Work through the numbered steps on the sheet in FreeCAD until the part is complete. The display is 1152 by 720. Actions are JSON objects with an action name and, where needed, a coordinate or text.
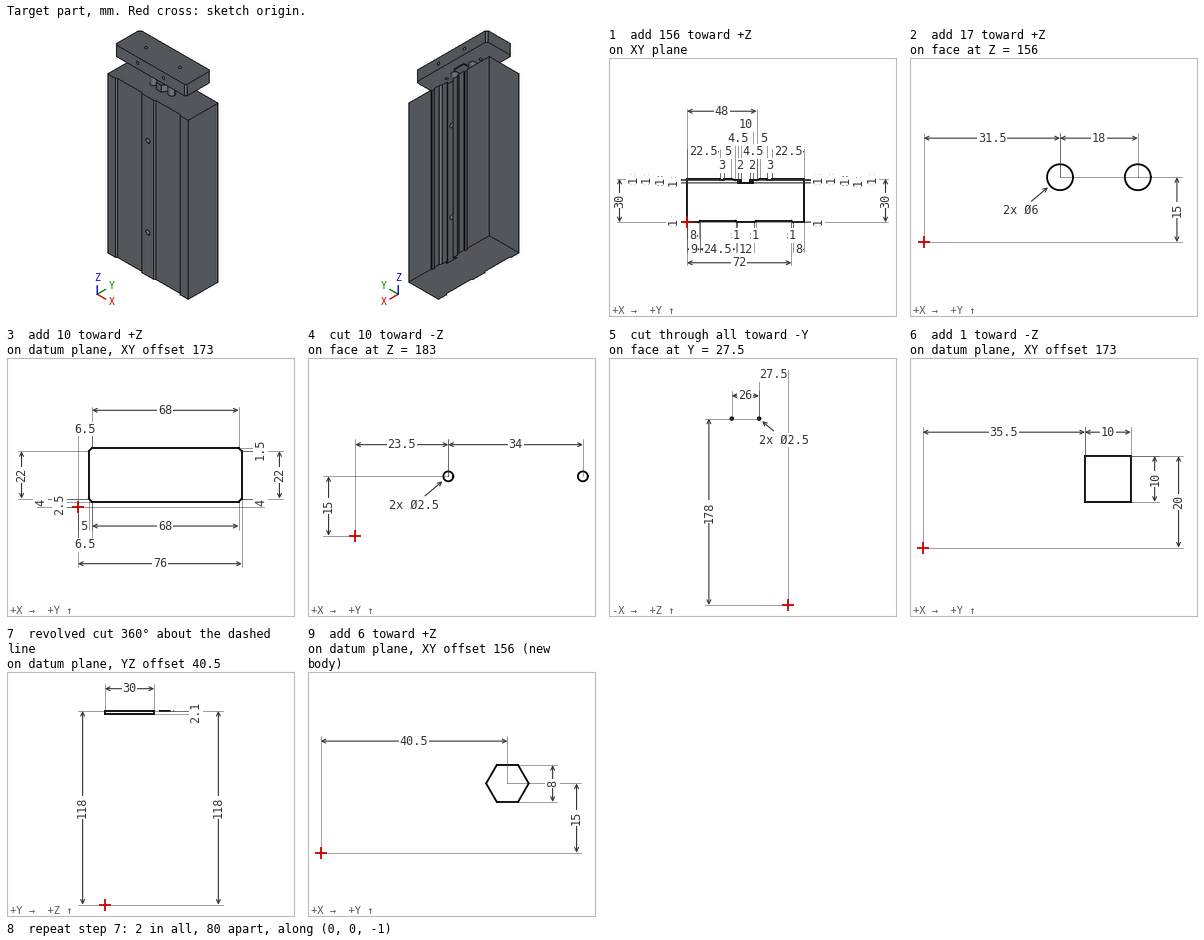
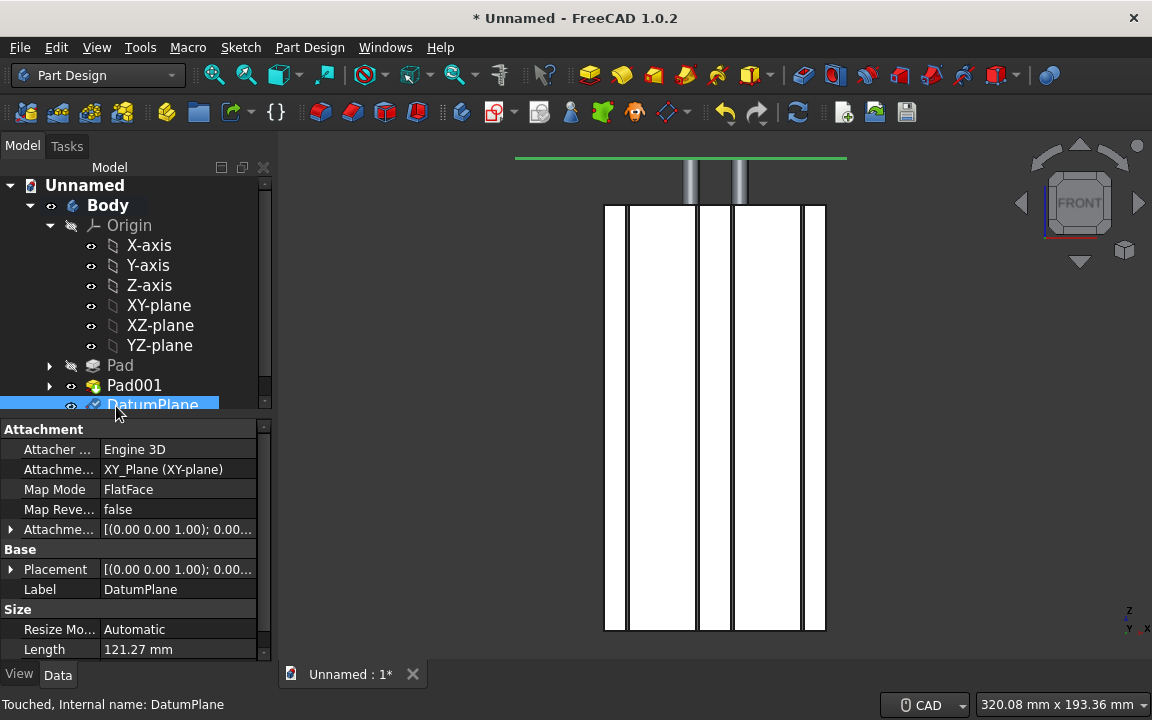
{"action": "left_click", "coordinate": [494, 112]}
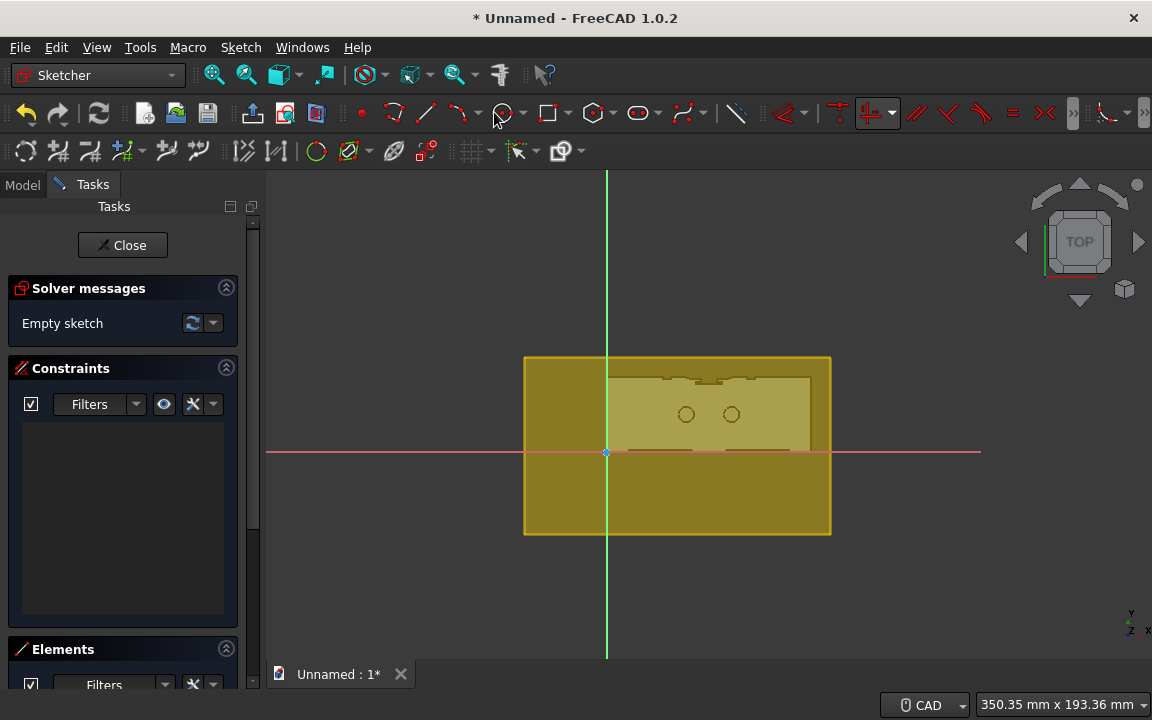
{"action": "scroll", "coordinate": [739, 420], "scroll_direction": "up", "scroll_amount": 5}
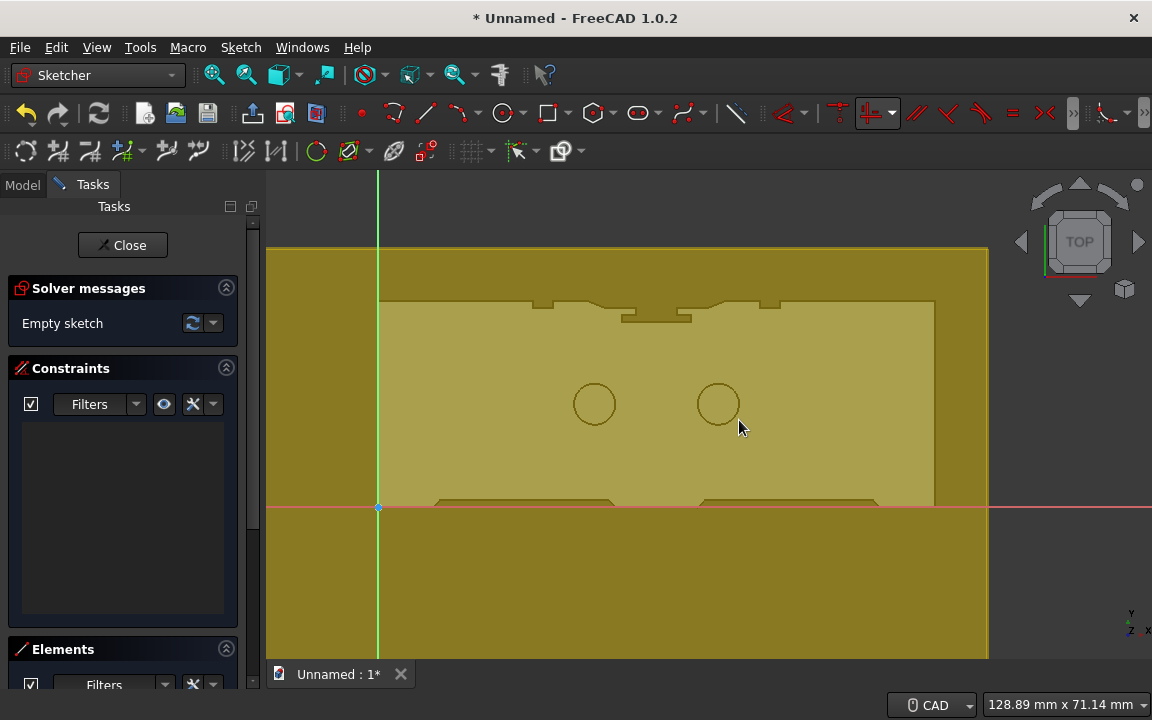
{"action": "left_click", "coordinate": [394, 114]}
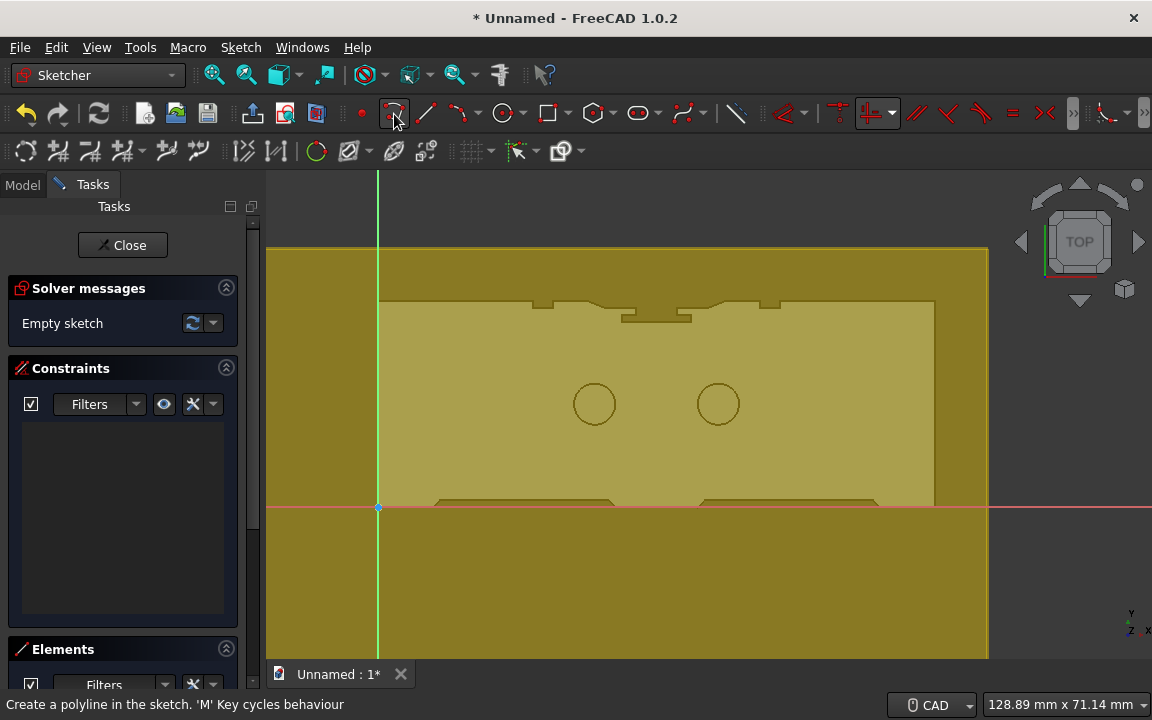
{"action": "left_click", "coordinate": [412, 480]}
{"action": "left_click", "coordinate": [423, 490]}
{"action": "left_click", "coordinate": [890, 490]}
{"action": "left_click", "coordinate": [901, 480]}
{"action": "left_click", "coordinate": [901, 329]}
{"action": "left_click", "coordinate": [890, 318]}
{"action": "left_click", "coordinate": [423, 318]}
{"action": "left_click", "coordinate": [412, 329]}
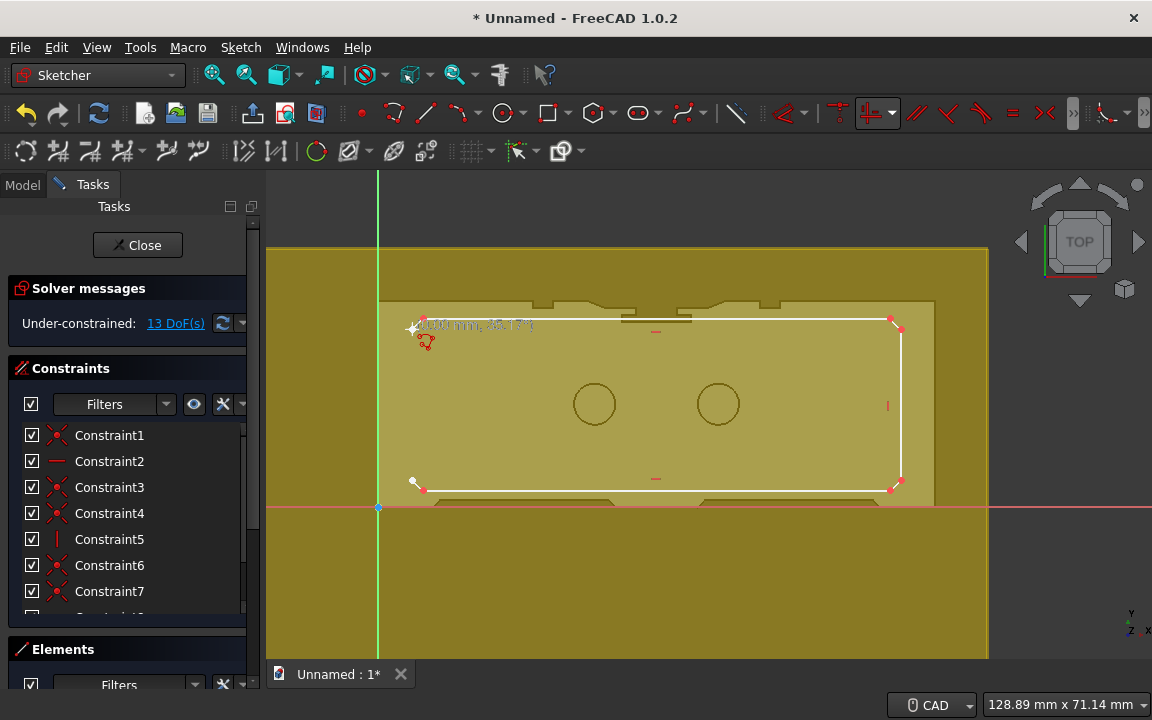
{"action": "scroll", "coordinate": [412, 480], "scroll_direction": "up", "scroll_amount": 4}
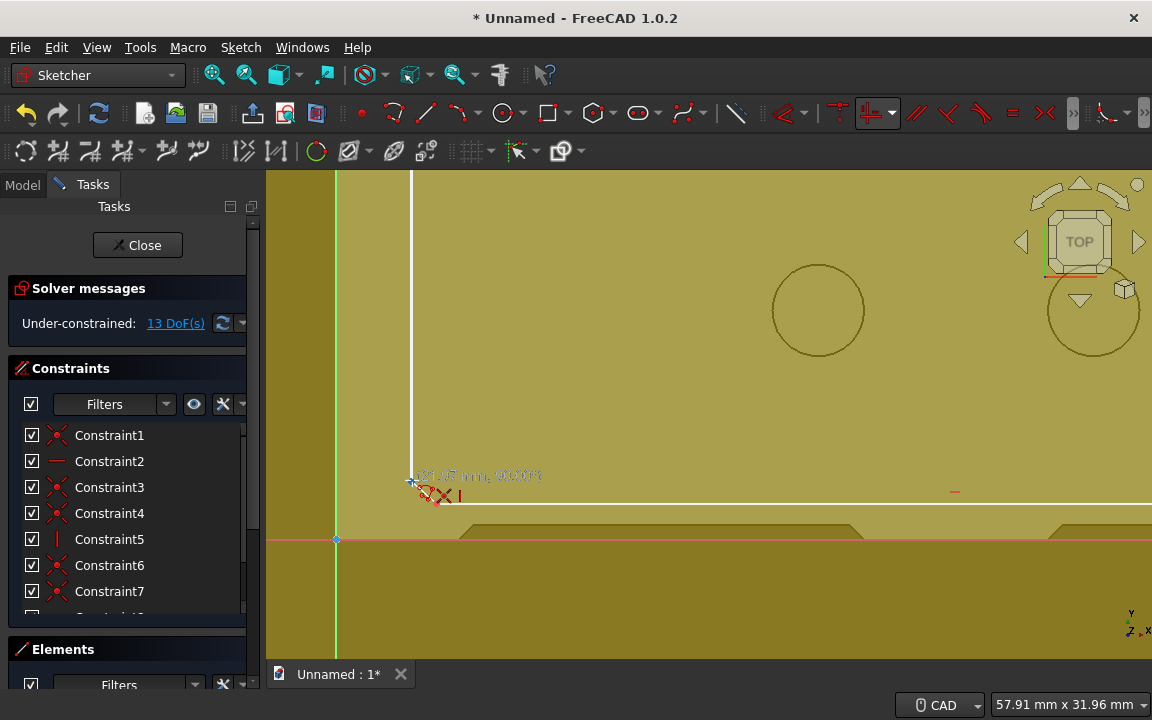
{"action": "left_click", "coordinate": [412, 481]}
{"action": "key", "text": "Escape"}
{"action": "key", "text": "Escape"}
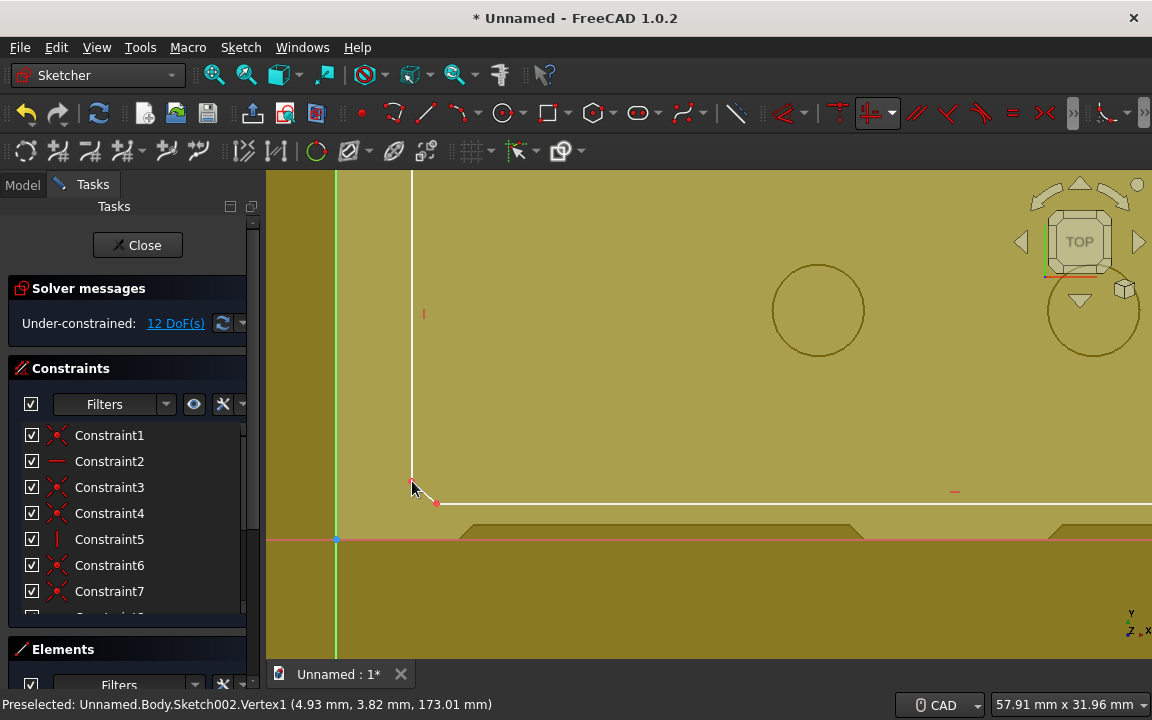
{"action": "left_click", "coordinate": [784, 114]}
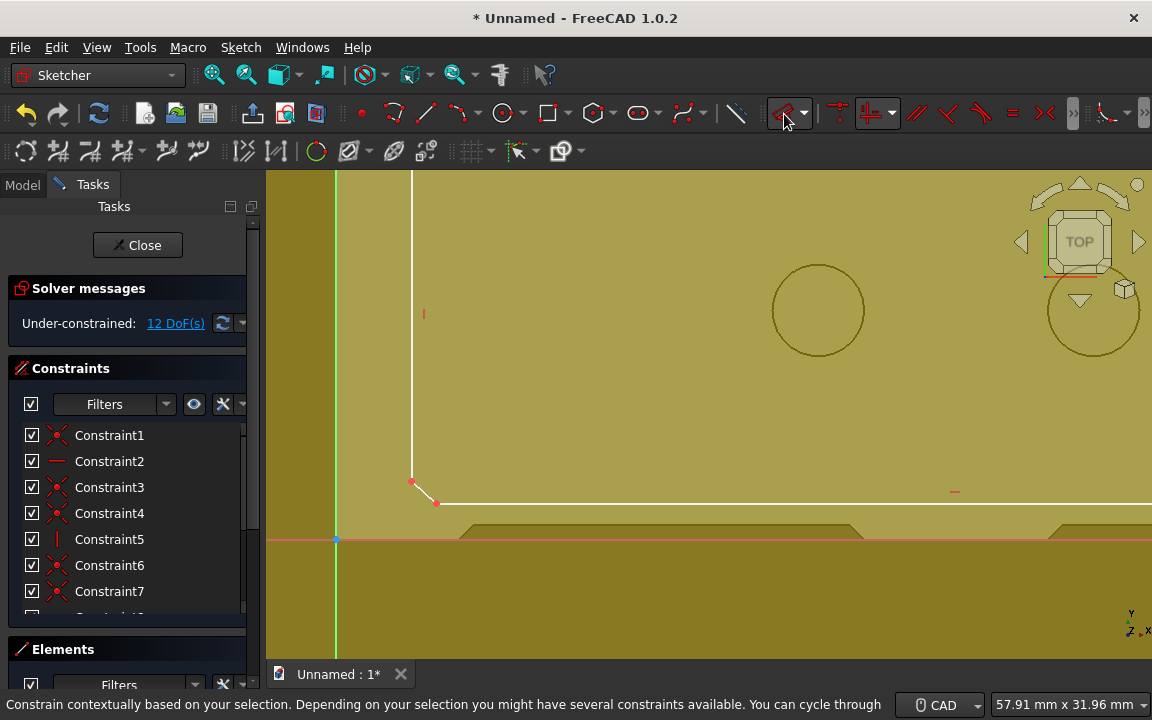
{"action": "left_click", "coordinate": [748, 504]}
{"action": "left_click", "coordinate": [712, 470]}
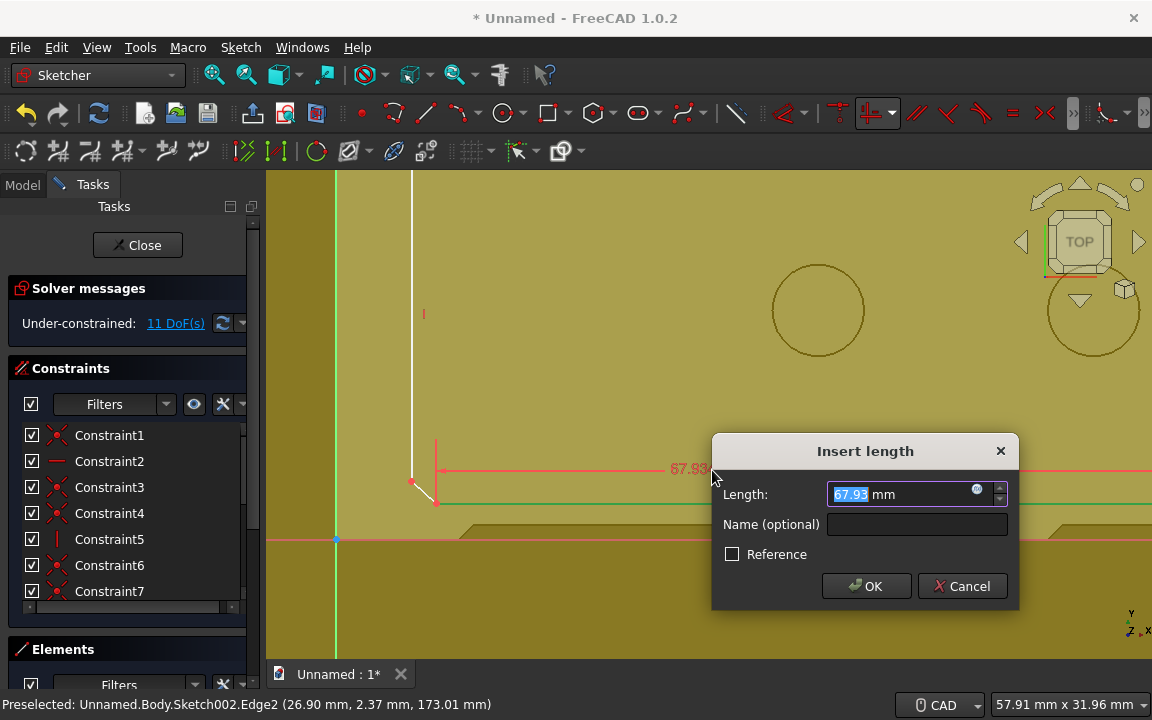
{"action": "type", "text": "68"}
{"action": "key", "text": "Return"}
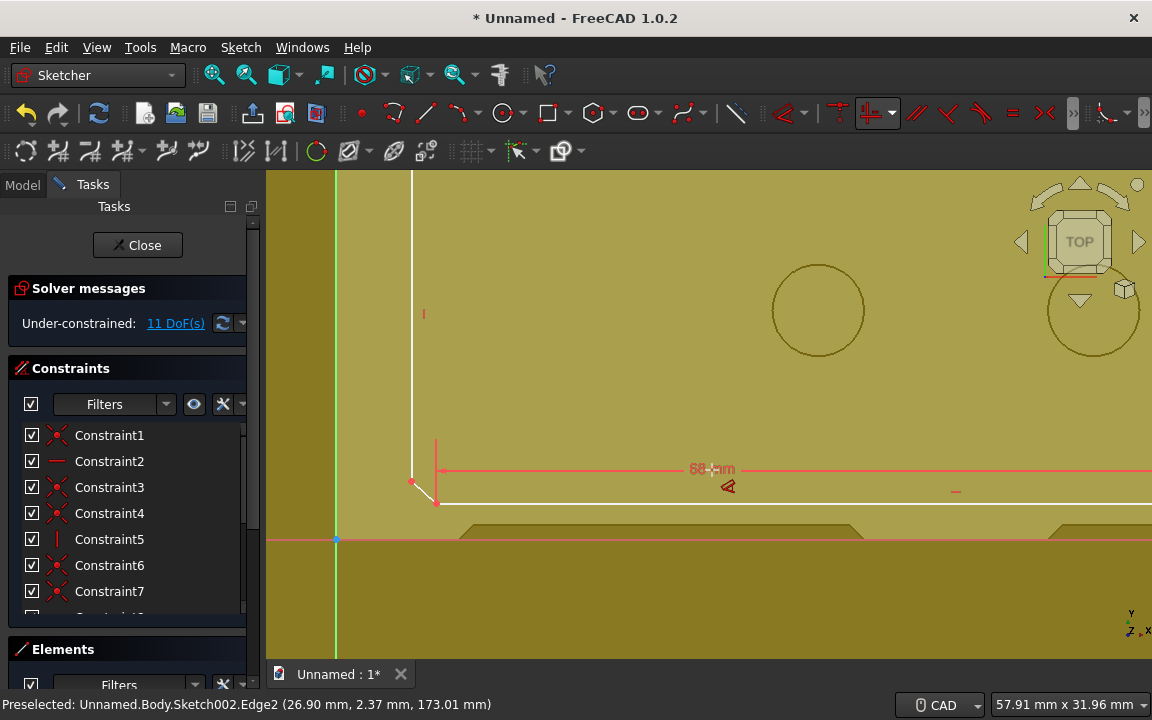
{"action": "scroll", "coordinate": [414, 484], "scroll_direction": "down", "scroll_amount": 4}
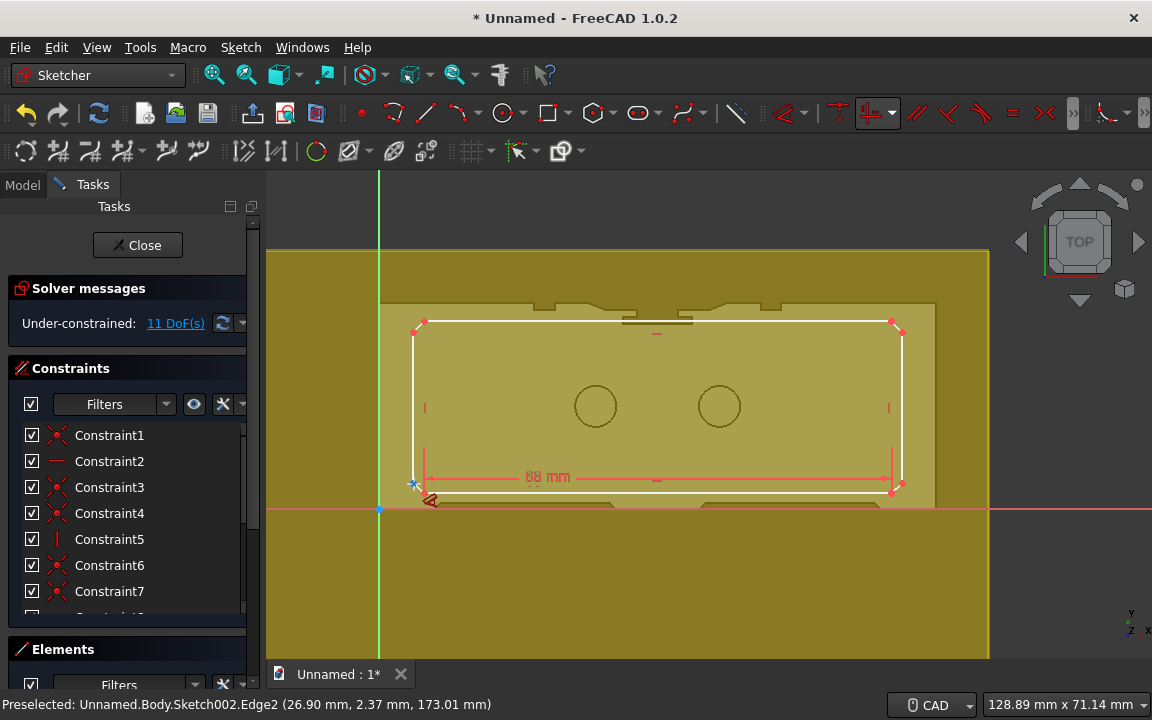
{"action": "left_click", "coordinate": [902, 438]}
{"action": "left_click", "coordinate": [936, 408]}